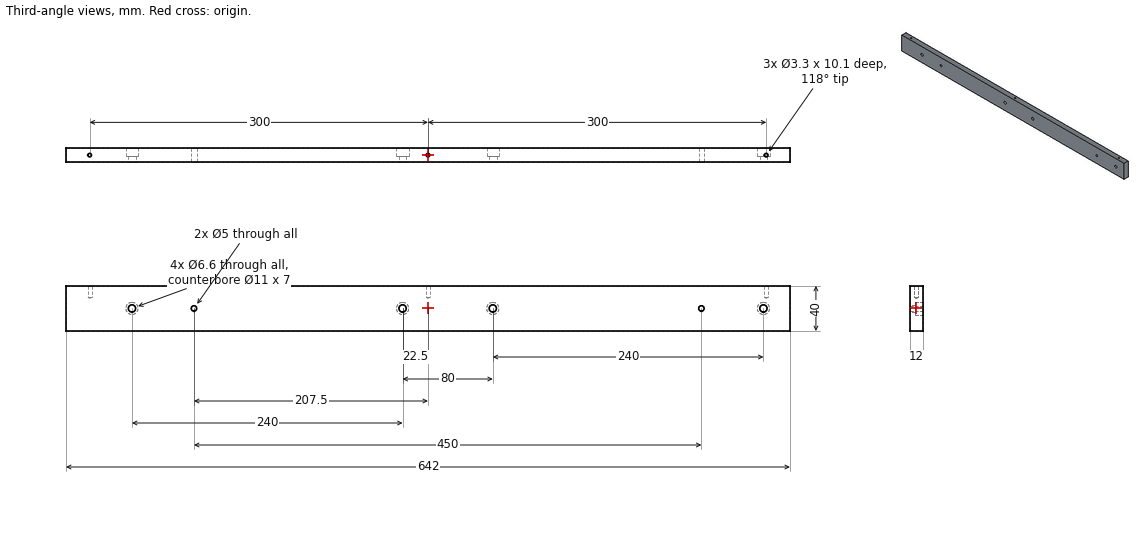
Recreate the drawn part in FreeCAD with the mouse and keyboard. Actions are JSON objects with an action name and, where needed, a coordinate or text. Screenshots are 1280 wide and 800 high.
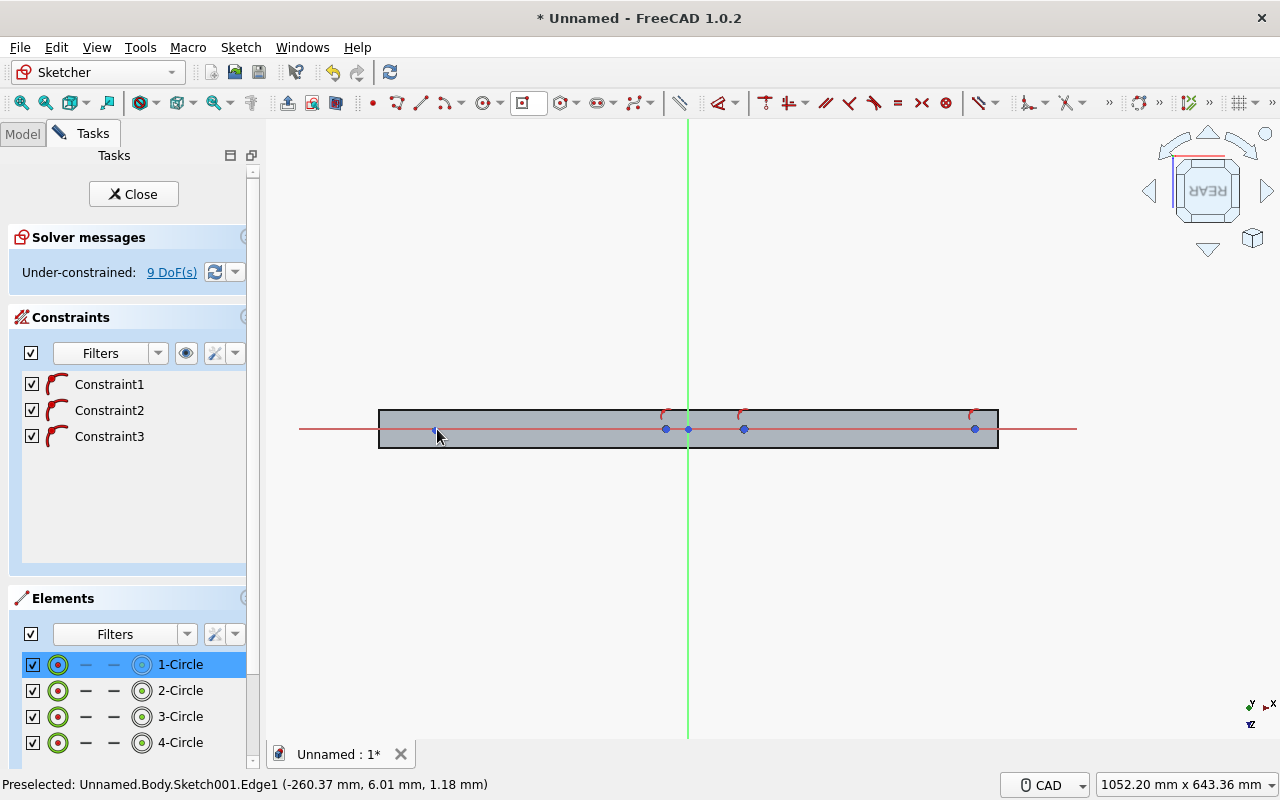
{"action": "scroll", "coordinate": [668, 427], "scroll_direction": "up", "scroll_amount": 9}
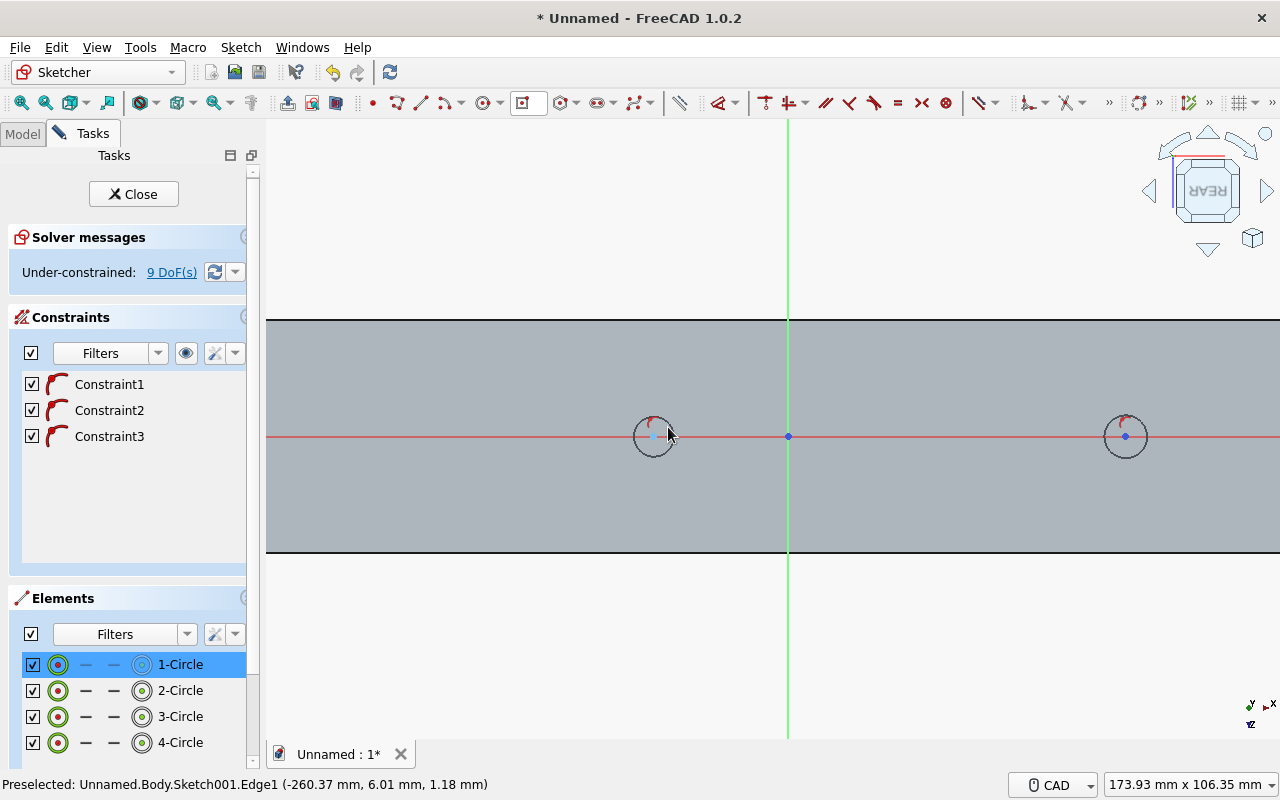
{"action": "left_click", "coordinate": [668, 423]}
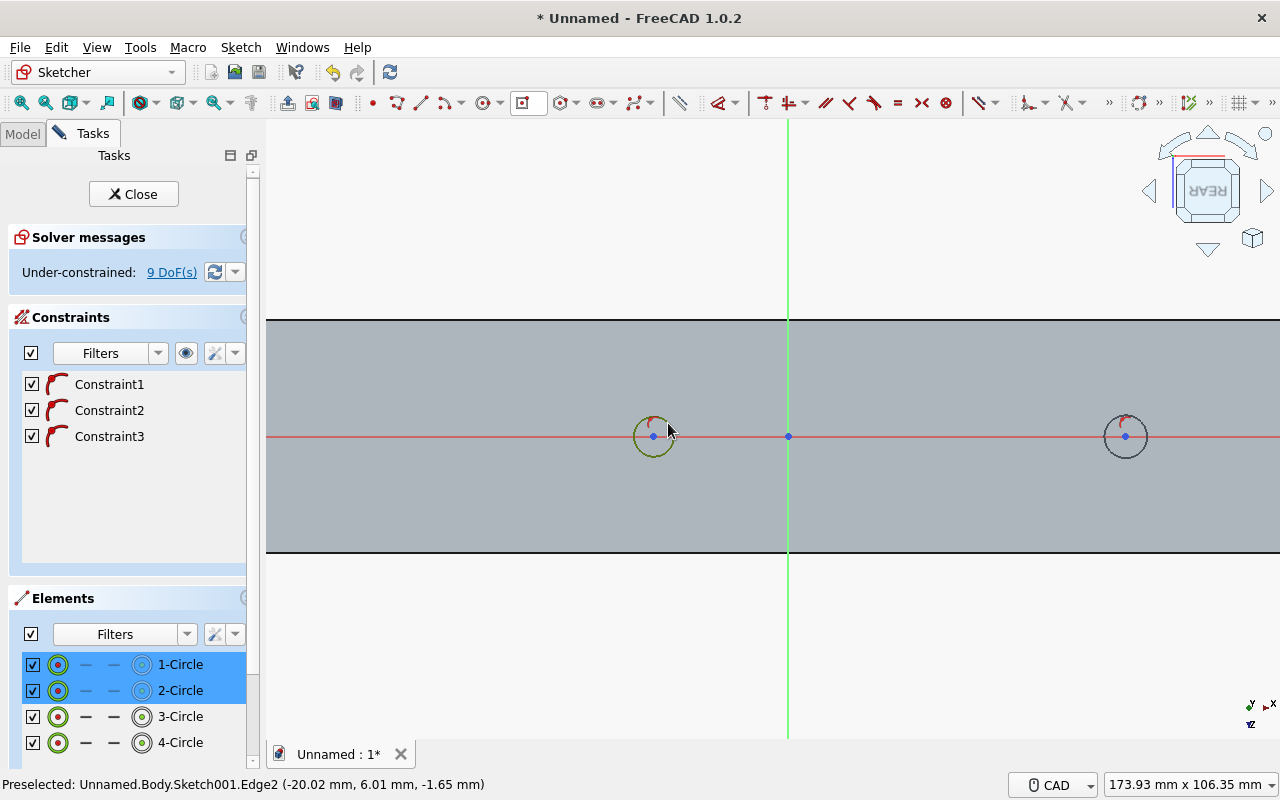
{"action": "left_click", "coordinate": [1111, 422]}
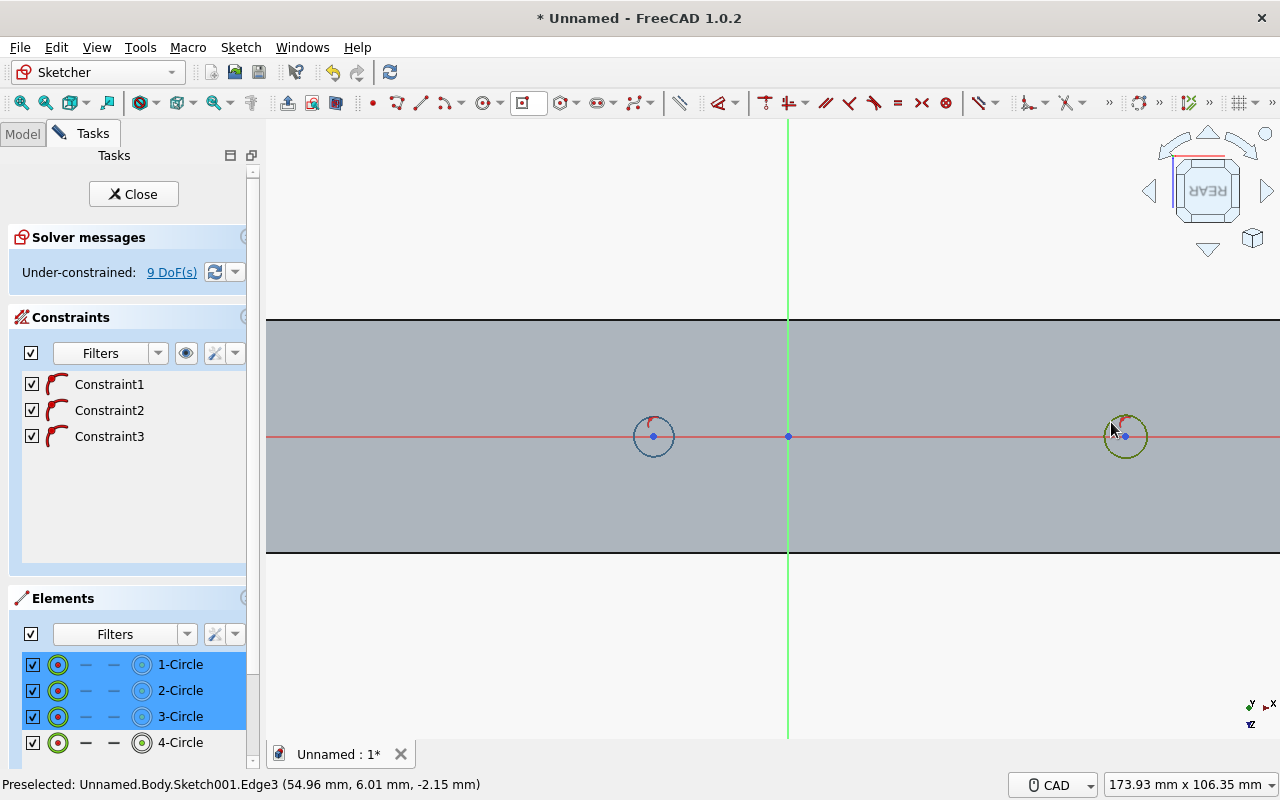
{"action": "scroll", "coordinate": [668, 427], "scroll_direction": "down", "scroll_amount": 9}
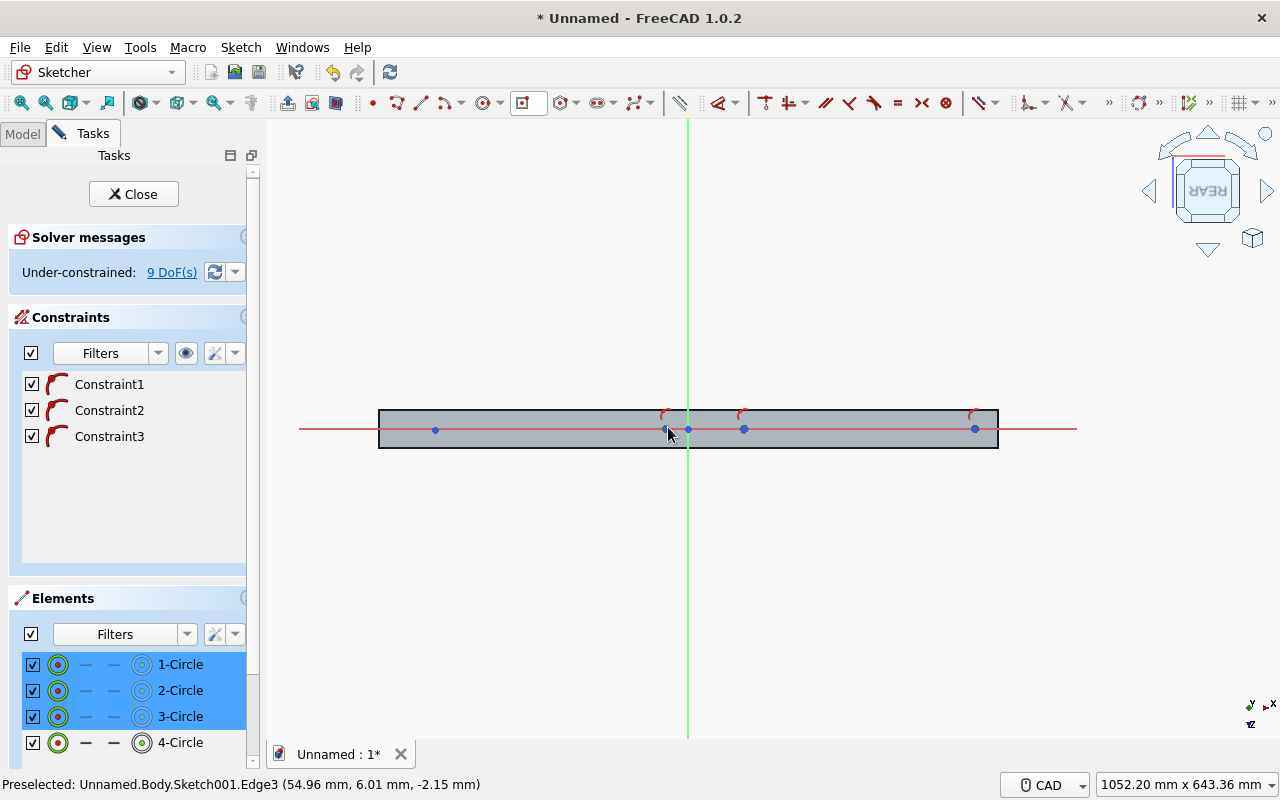
{"action": "scroll", "coordinate": [977, 427], "scroll_direction": "up", "scroll_amount": 9}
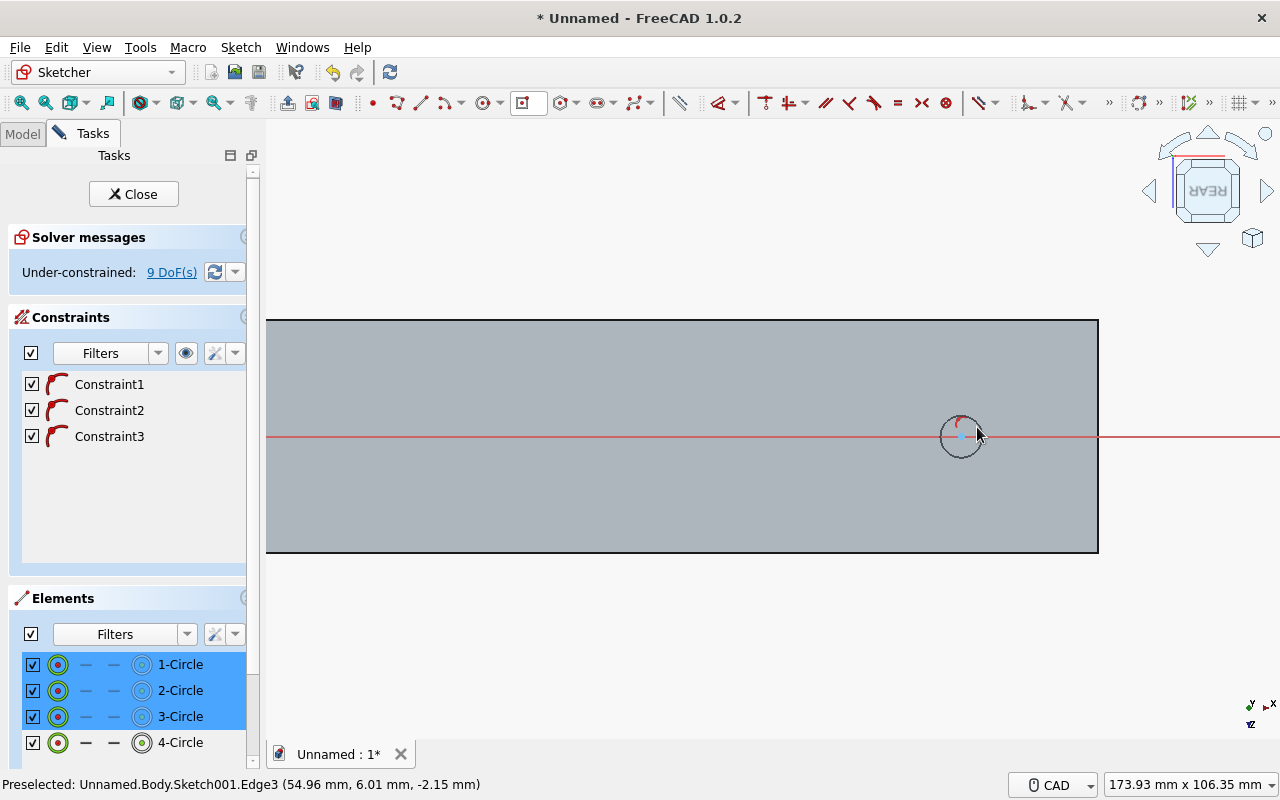
{"action": "left_click", "coordinate": [976, 422]}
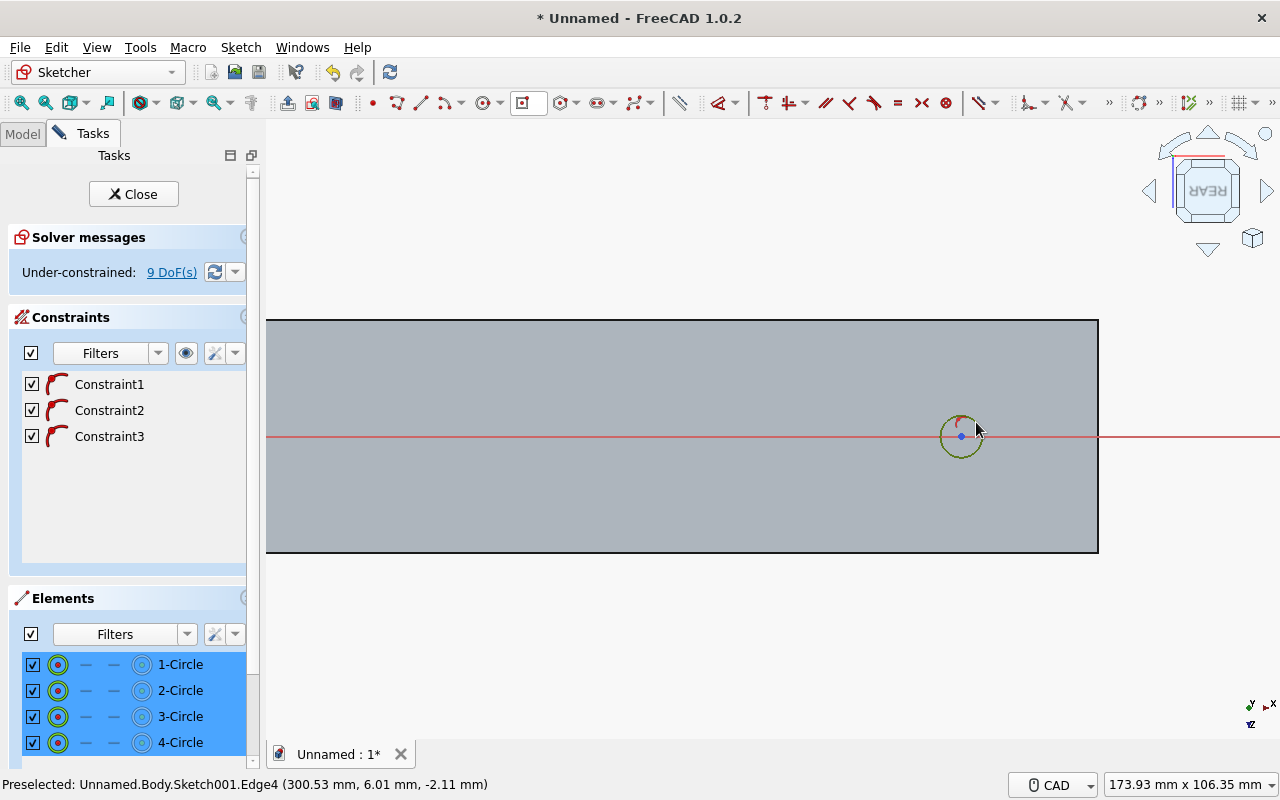
{"action": "left_click", "coordinate": [898, 104]}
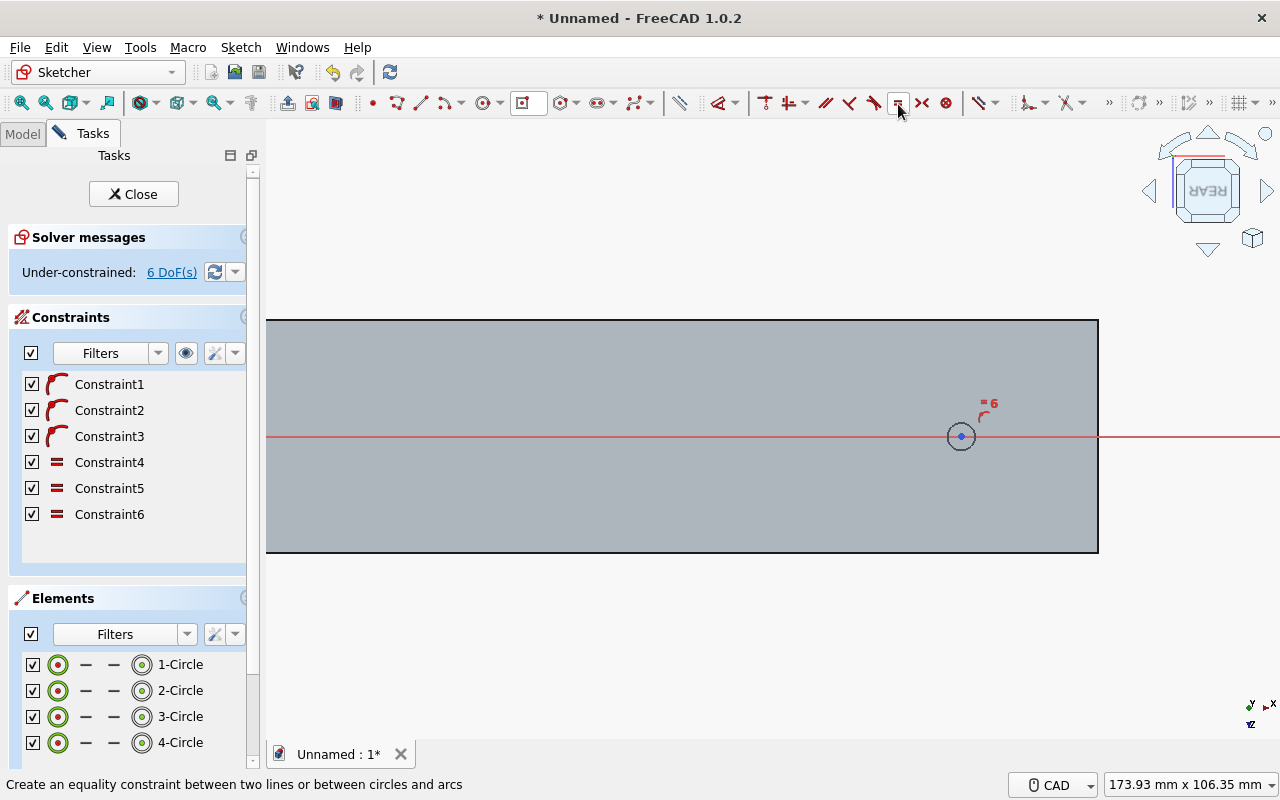
{"action": "scroll", "coordinate": [977, 427], "scroll_direction": "down", "scroll_amount": 9}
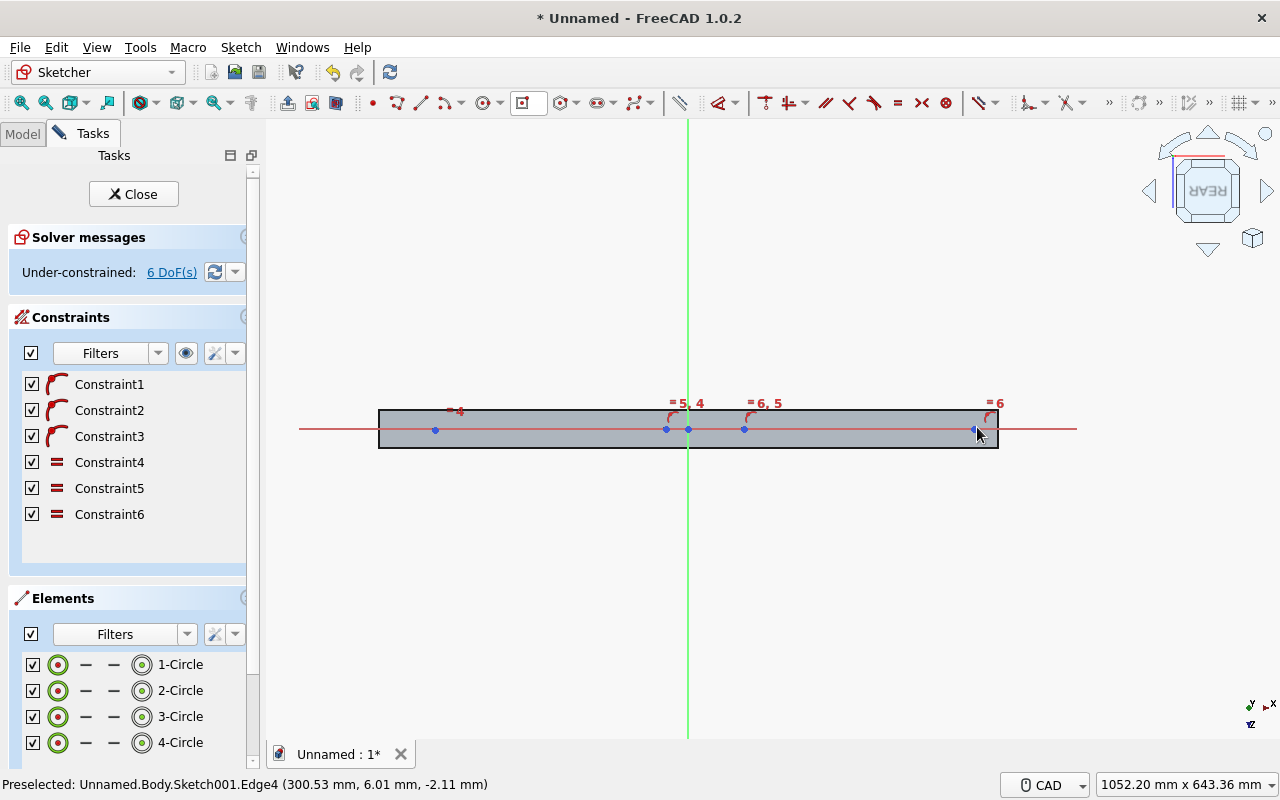
{"action": "left_click", "coordinate": [435, 430]}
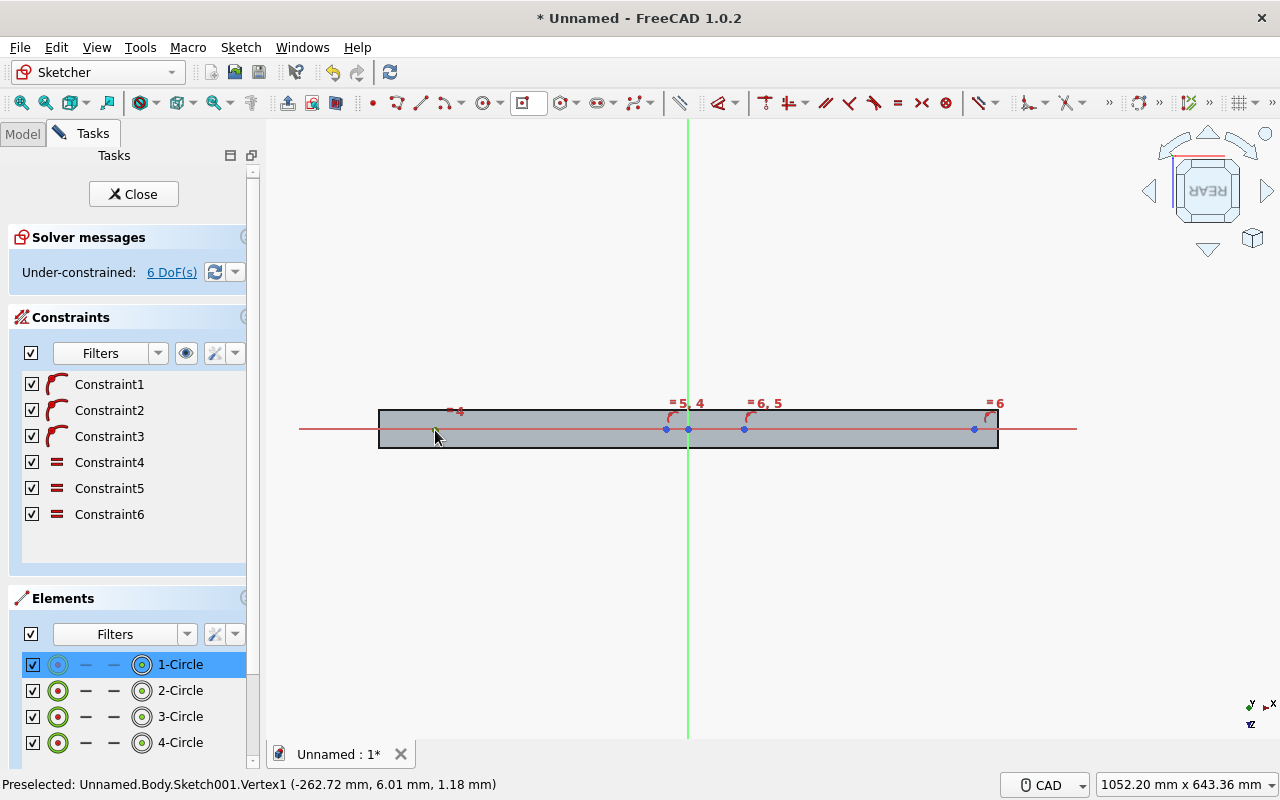
{"action": "left_click", "coordinate": [353, 429]}